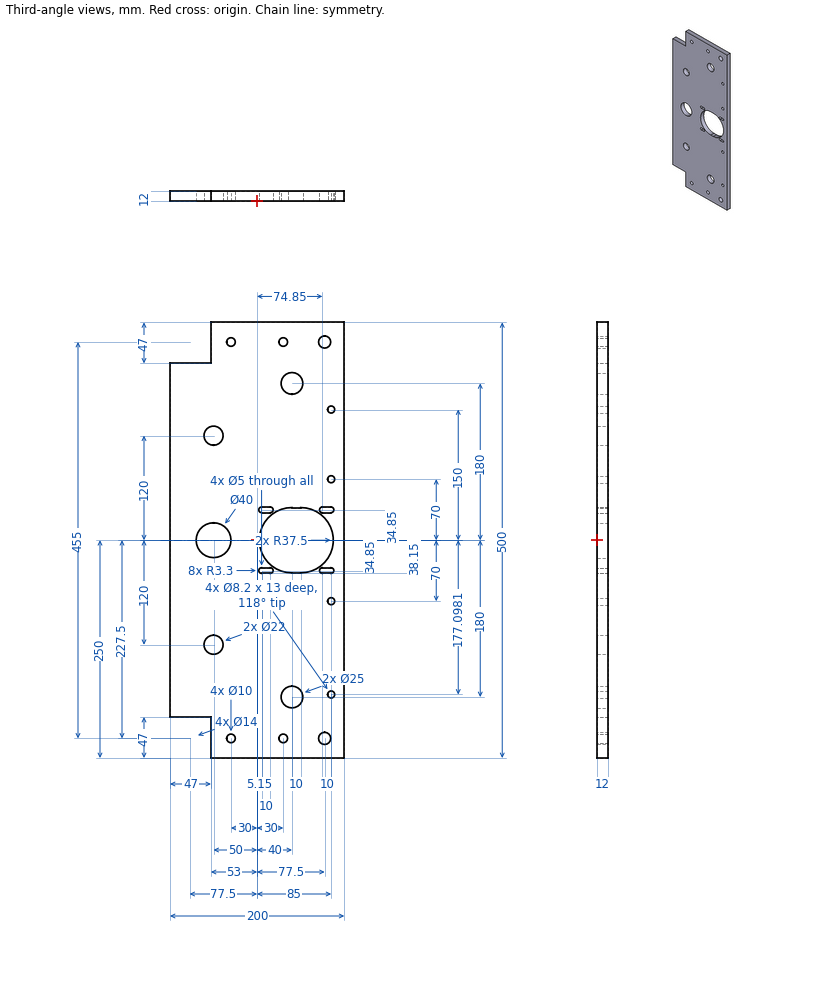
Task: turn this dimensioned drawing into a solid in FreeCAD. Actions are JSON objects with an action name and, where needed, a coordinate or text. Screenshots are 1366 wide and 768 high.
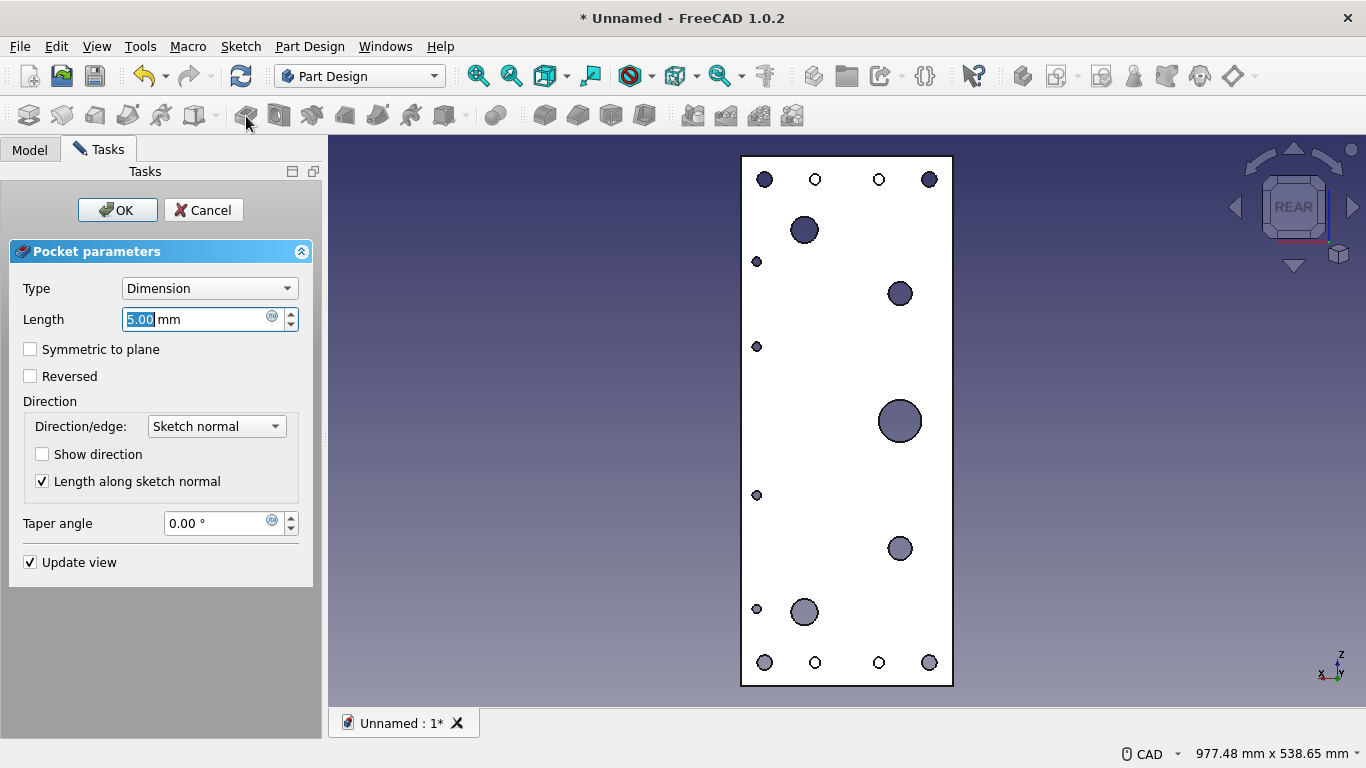
{"action": "left_click", "coordinate": [210, 288]}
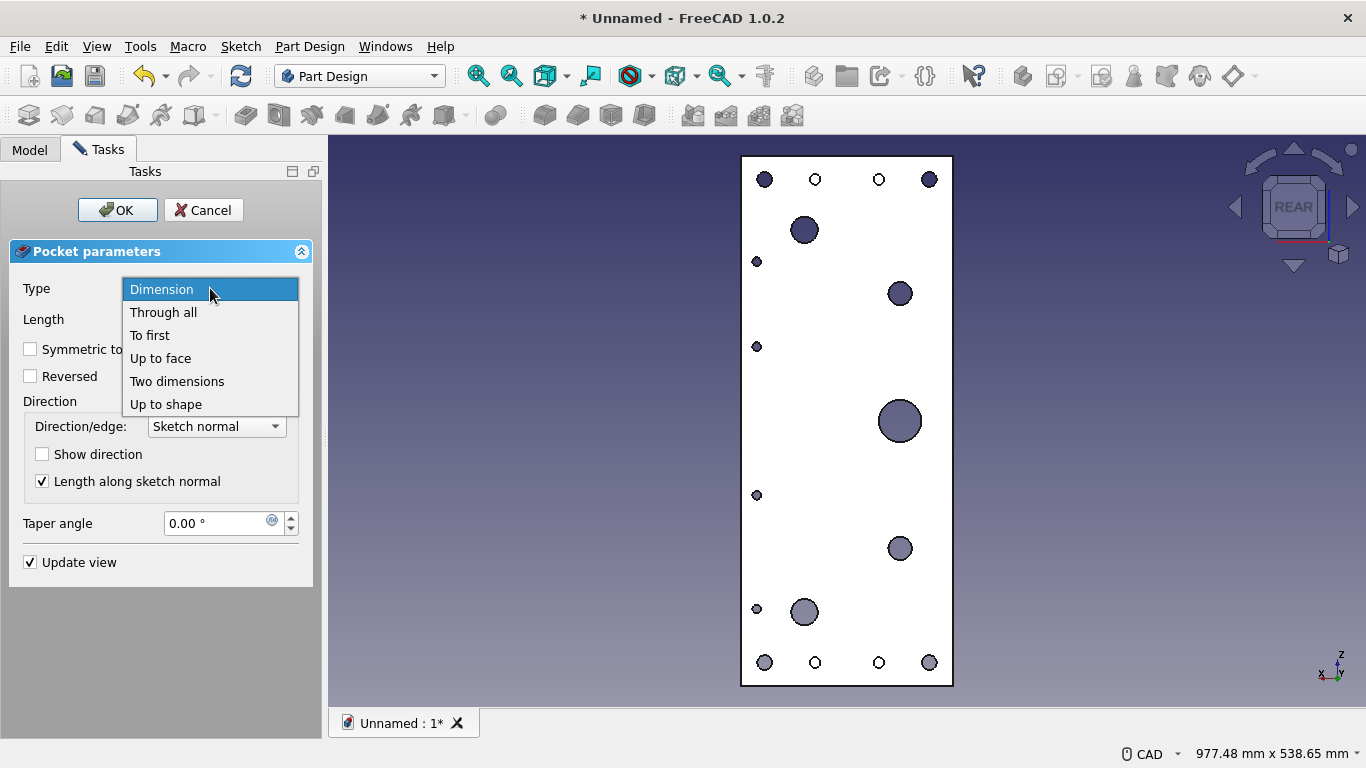
{"action": "left_click", "coordinate": [208, 312]}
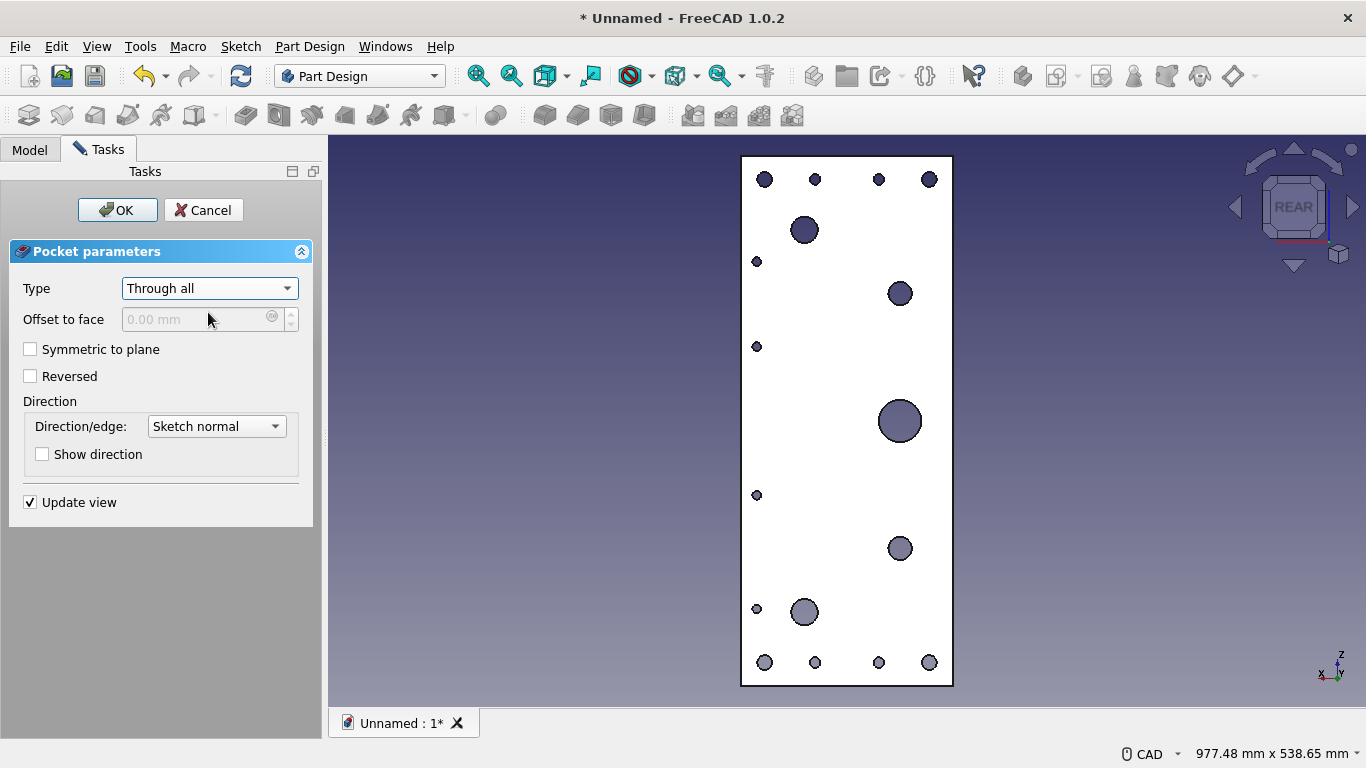
{"action": "left_click", "coordinate": [118, 210]}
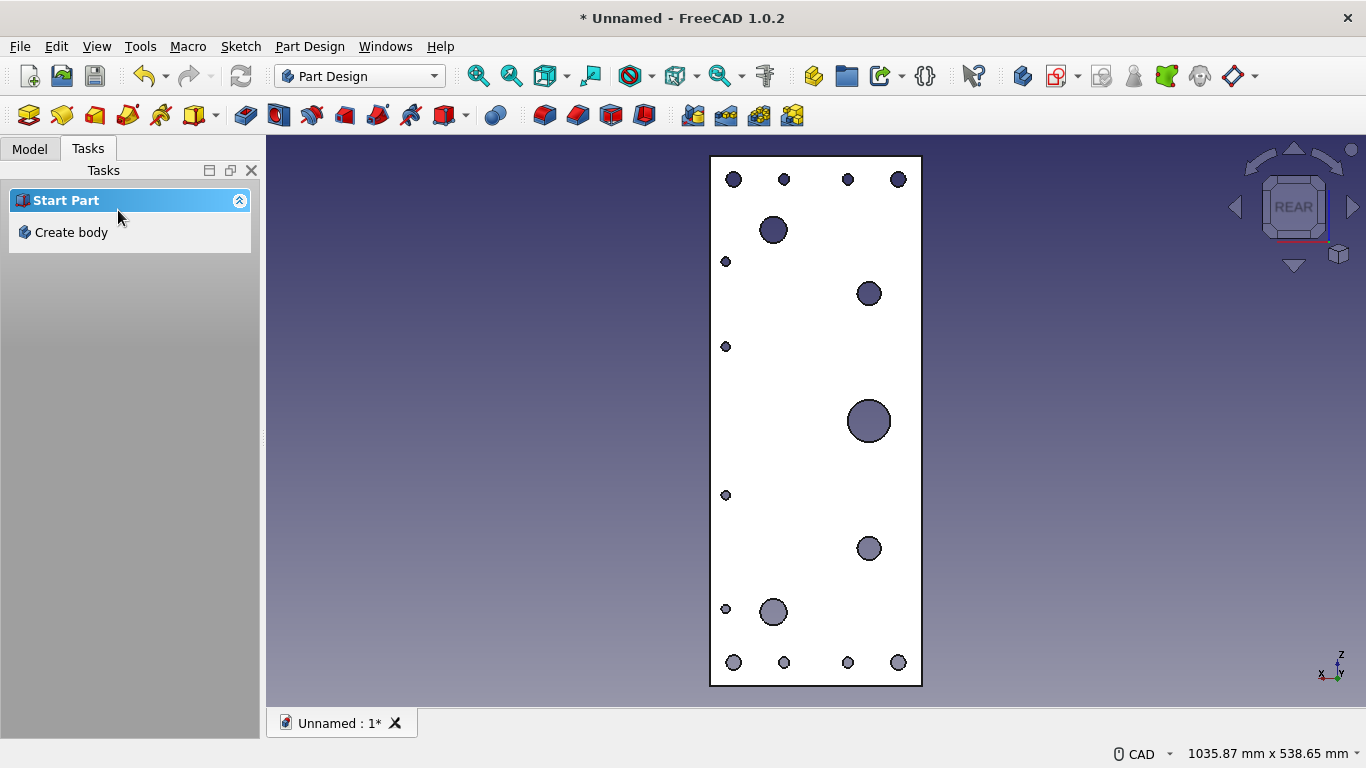
{"action": "left_click", "coordinate": [816, 496]}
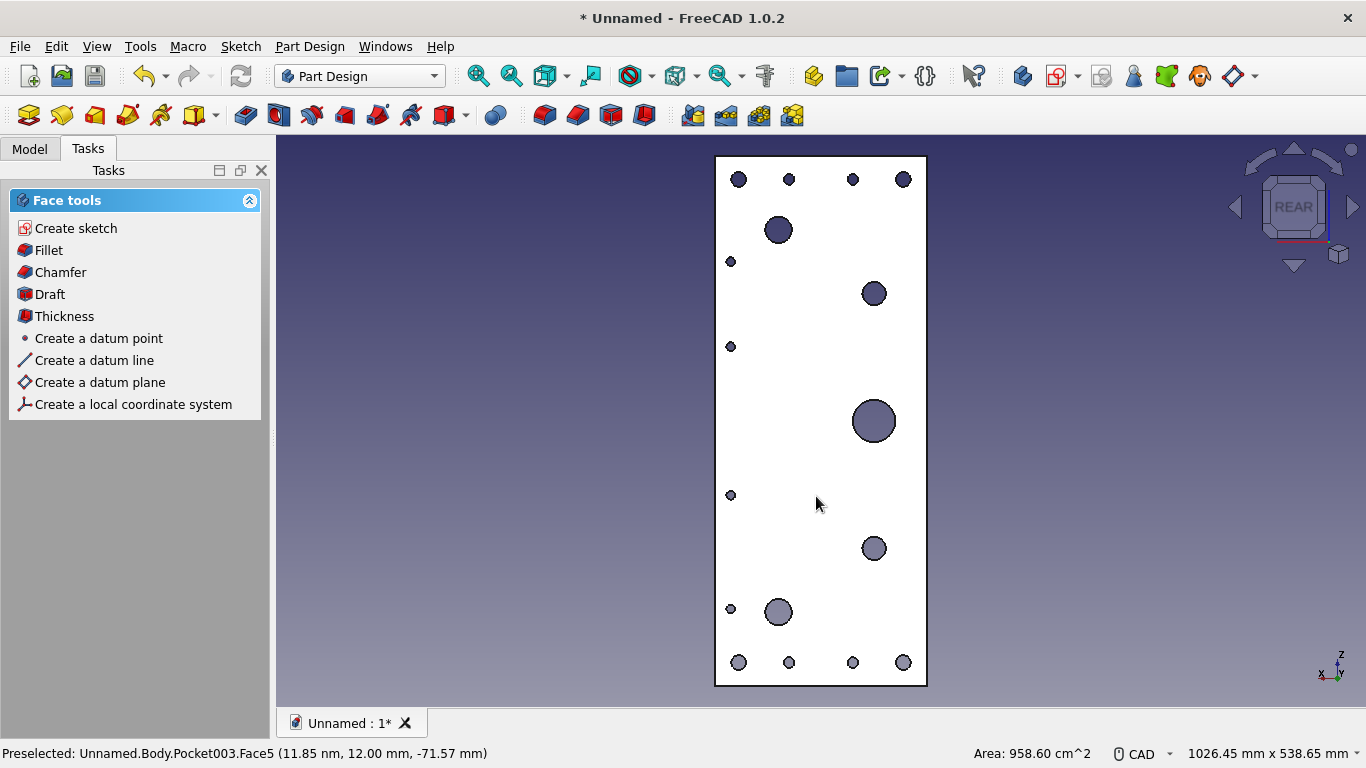
{"action": "left_click", "coordinate": [1056, 76]}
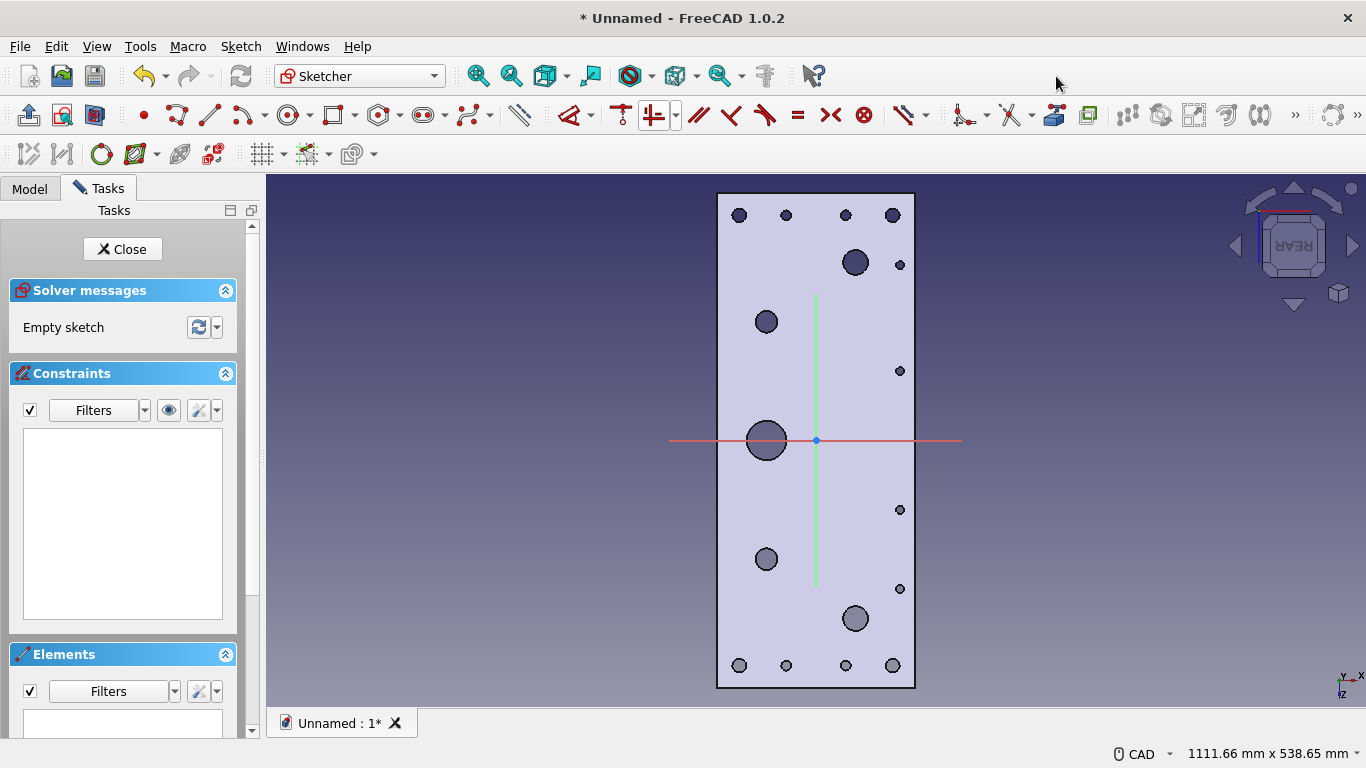
{"action": "scroll", "coordinate": [709, 441], "scroll_direction": "down", "scroll_amount": 2}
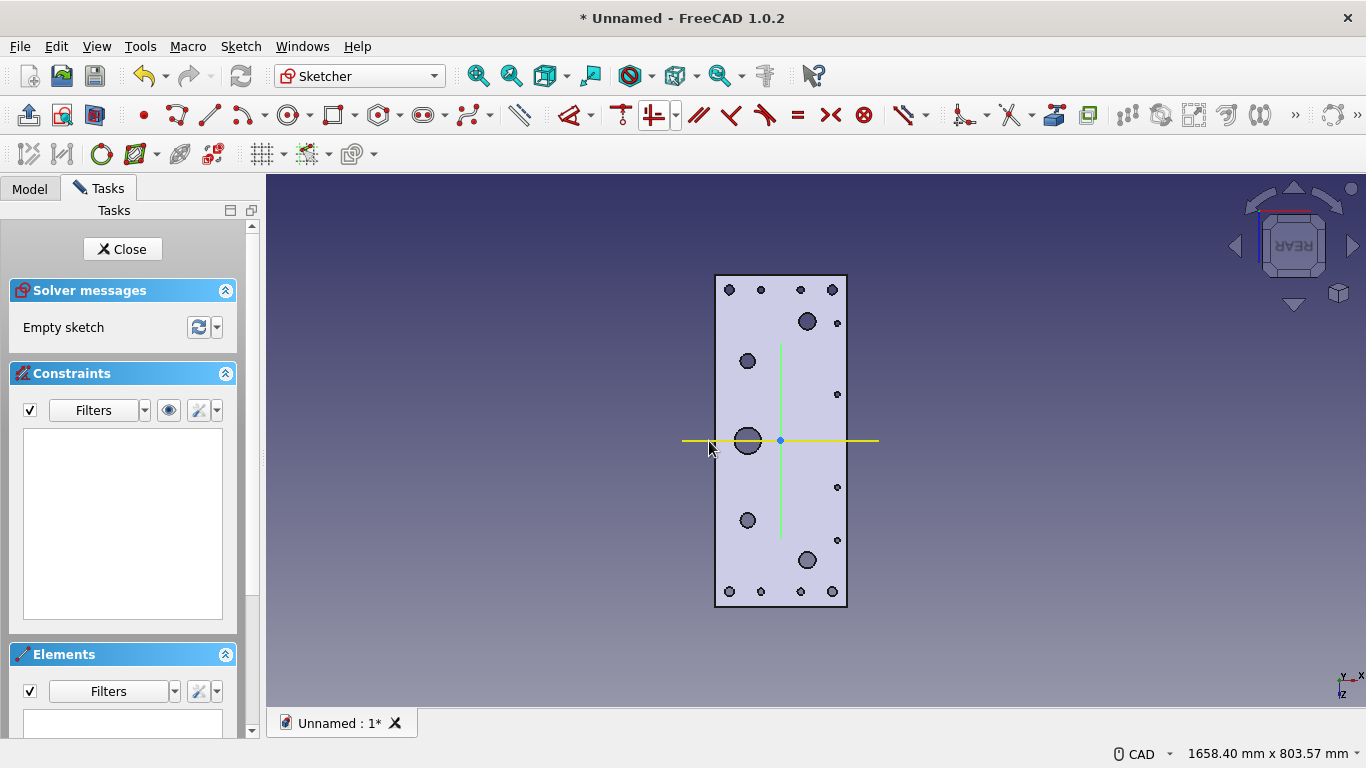
{"action": "left_click", "coordinate": [332, 116]}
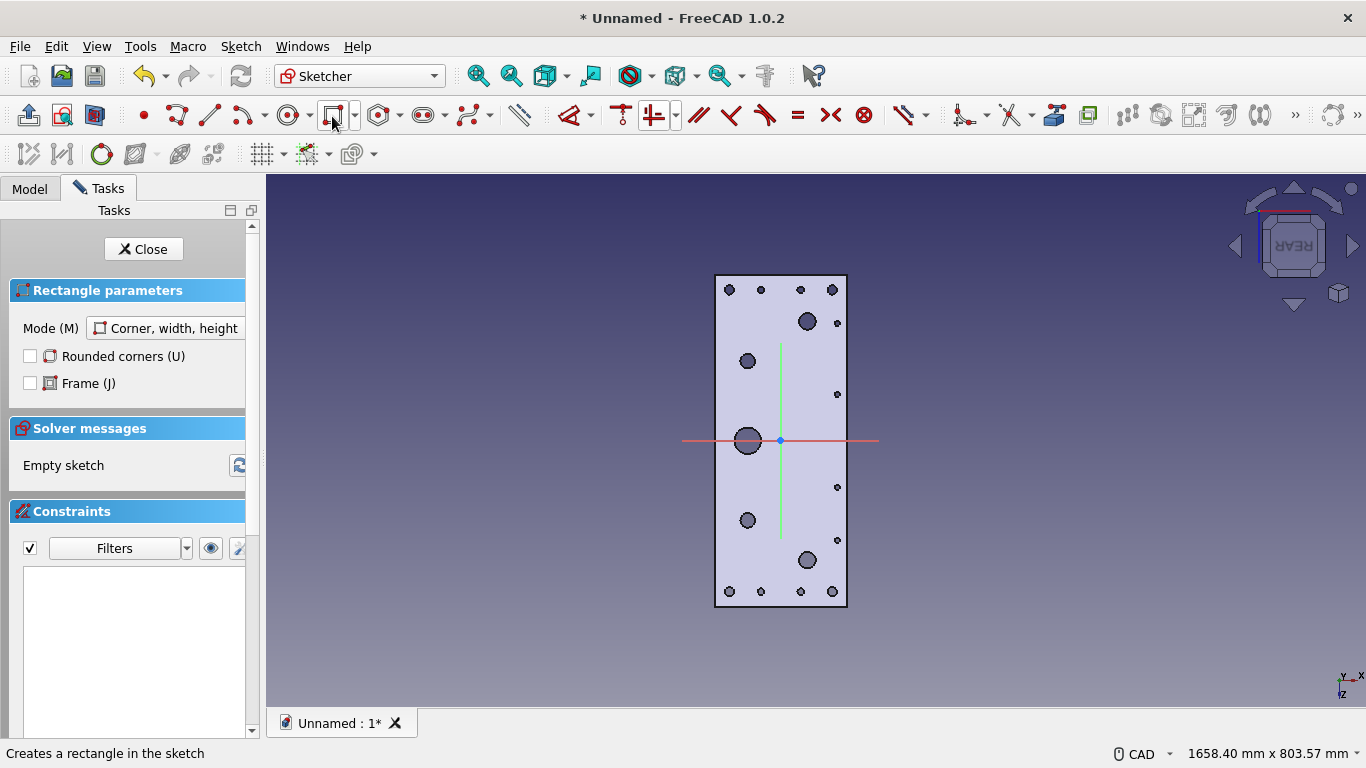
{"action": "left_click", "coordinate": [715, 275]}
{"action": "mouse_move", "coordinate": [746, 306]}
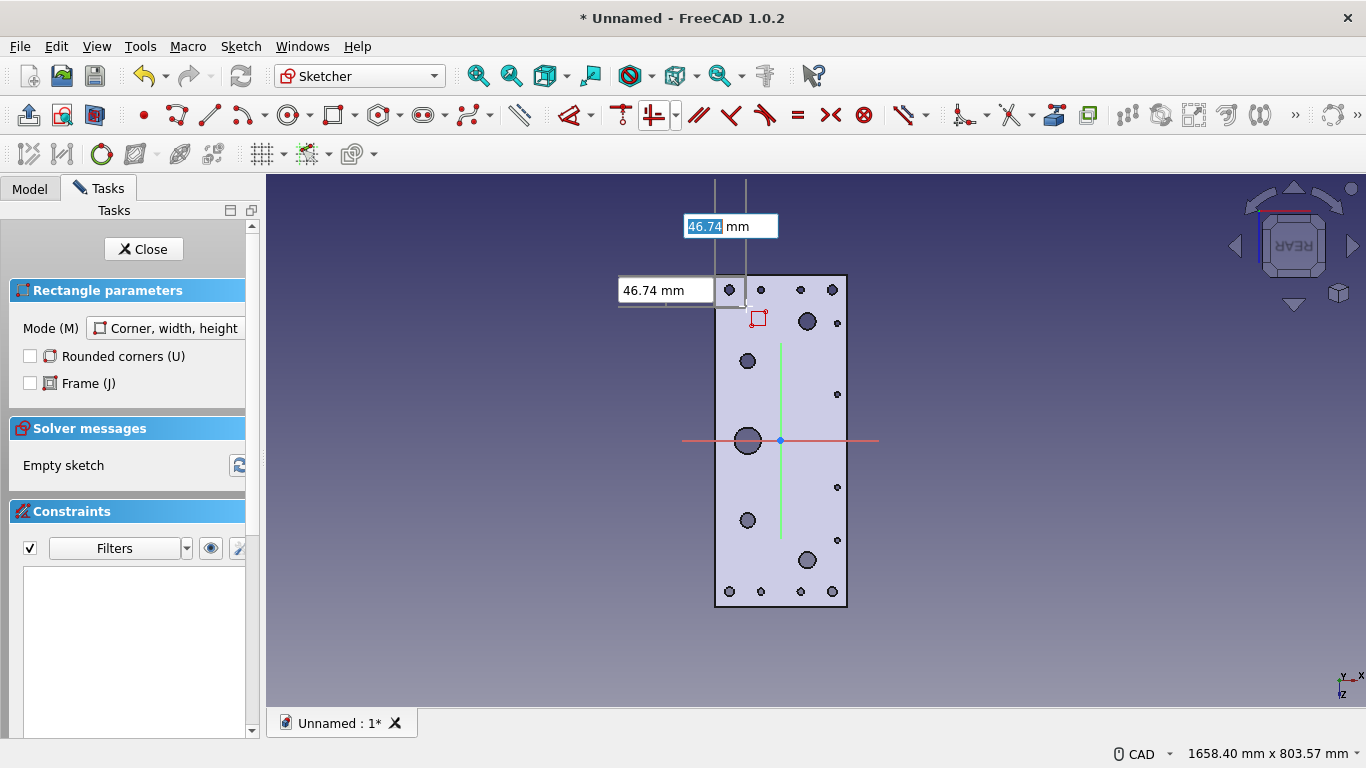
{"action": "type", "text": "47"}
{"action": "key", "text": "Tab"}
{"action": "type", "text": "47"}
{"action": "key", "text": "Return"}